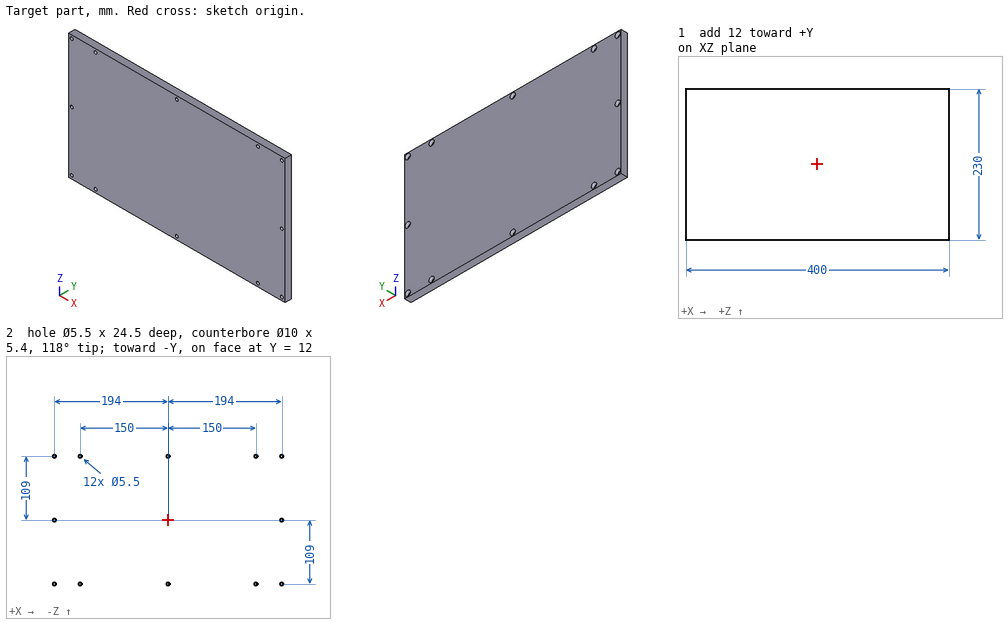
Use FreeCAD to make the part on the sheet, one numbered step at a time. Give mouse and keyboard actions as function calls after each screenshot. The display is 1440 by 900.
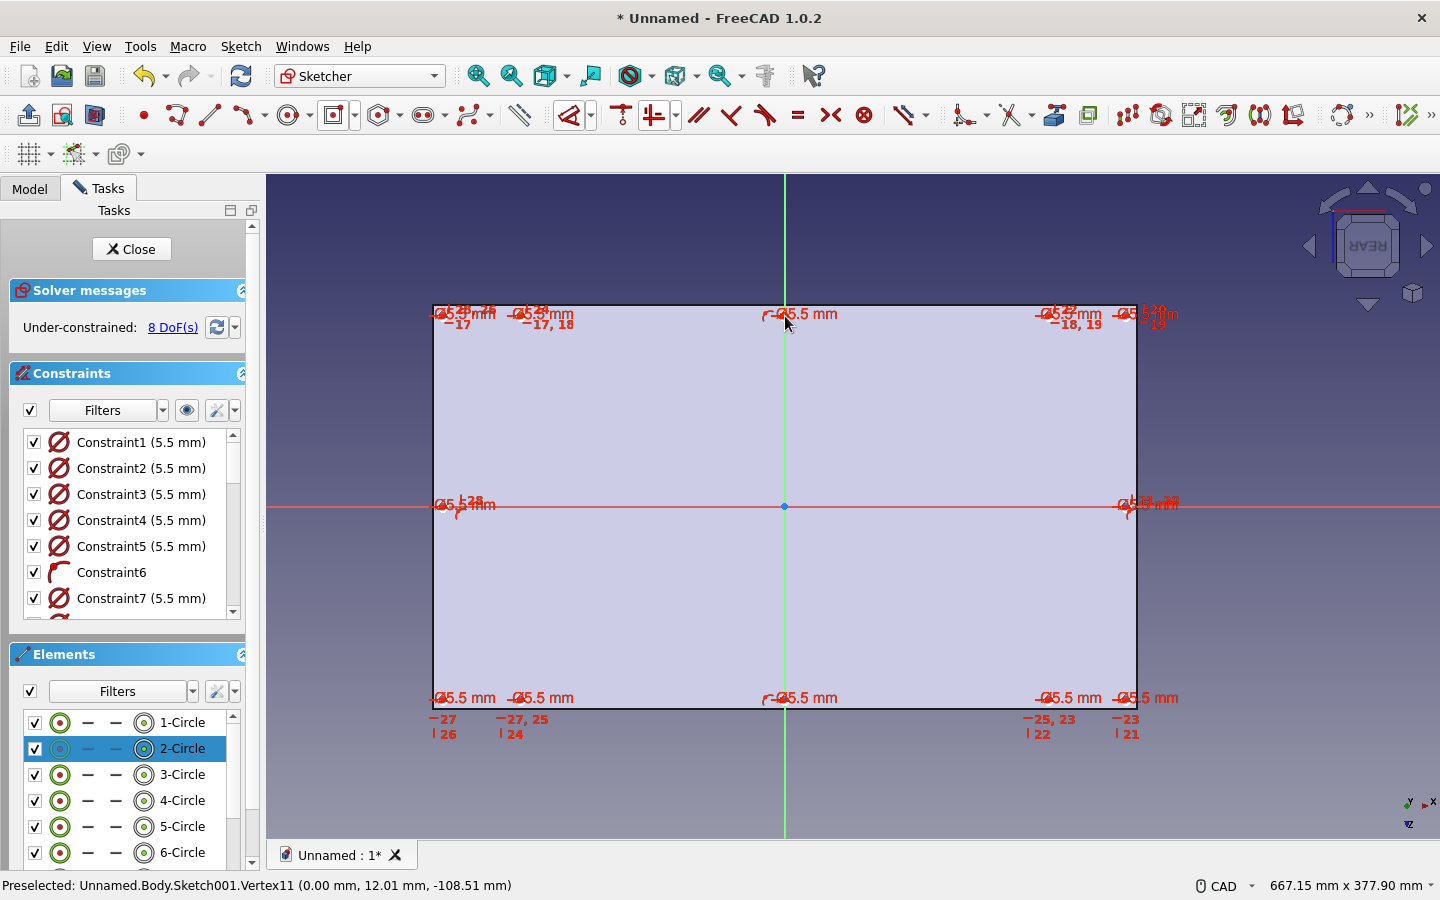
click(676, 116)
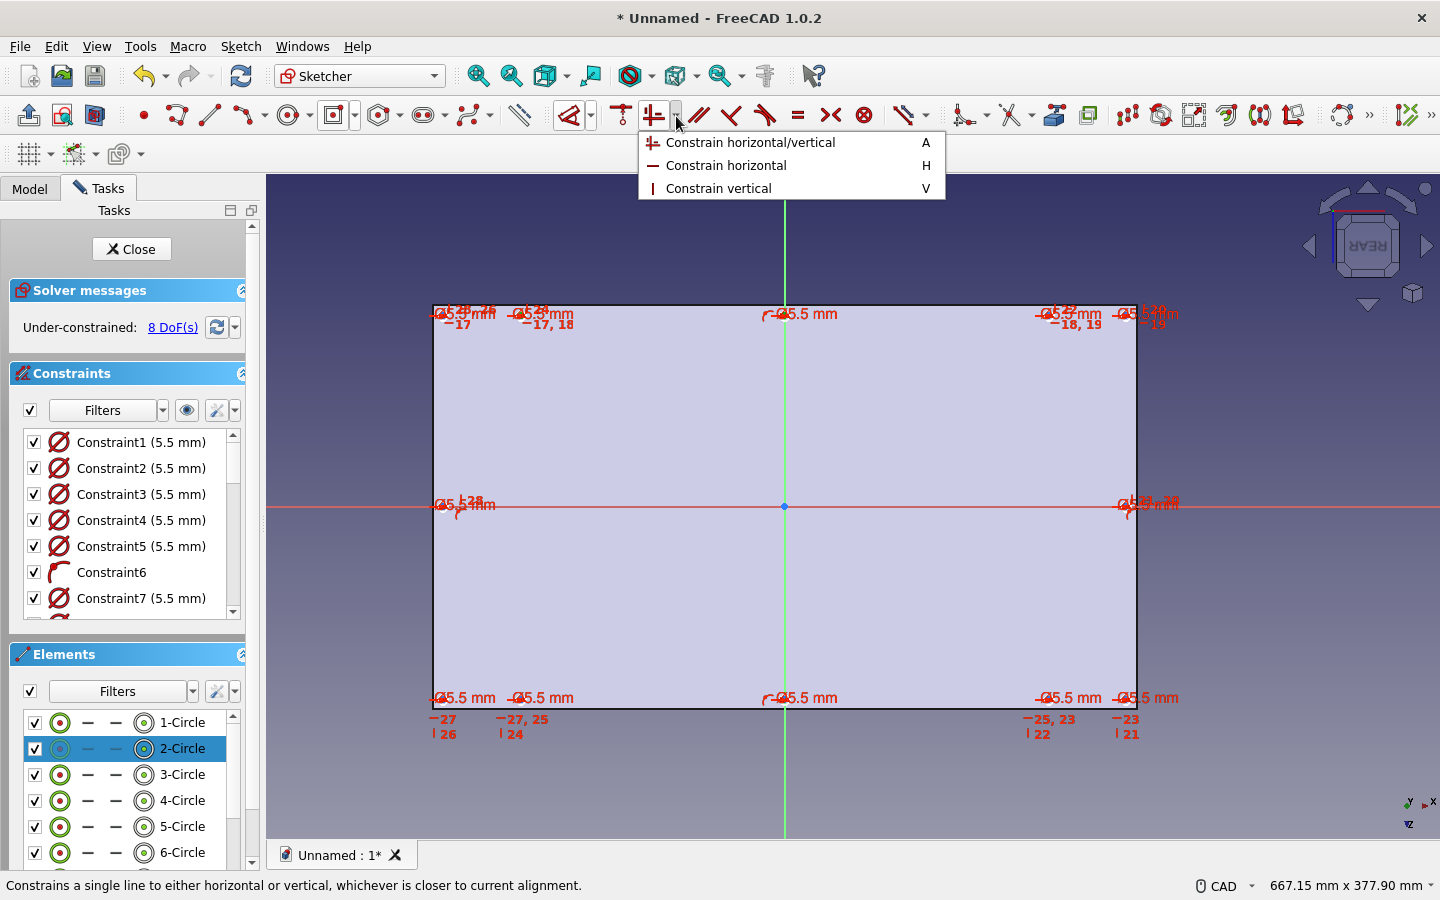
click(792, 166)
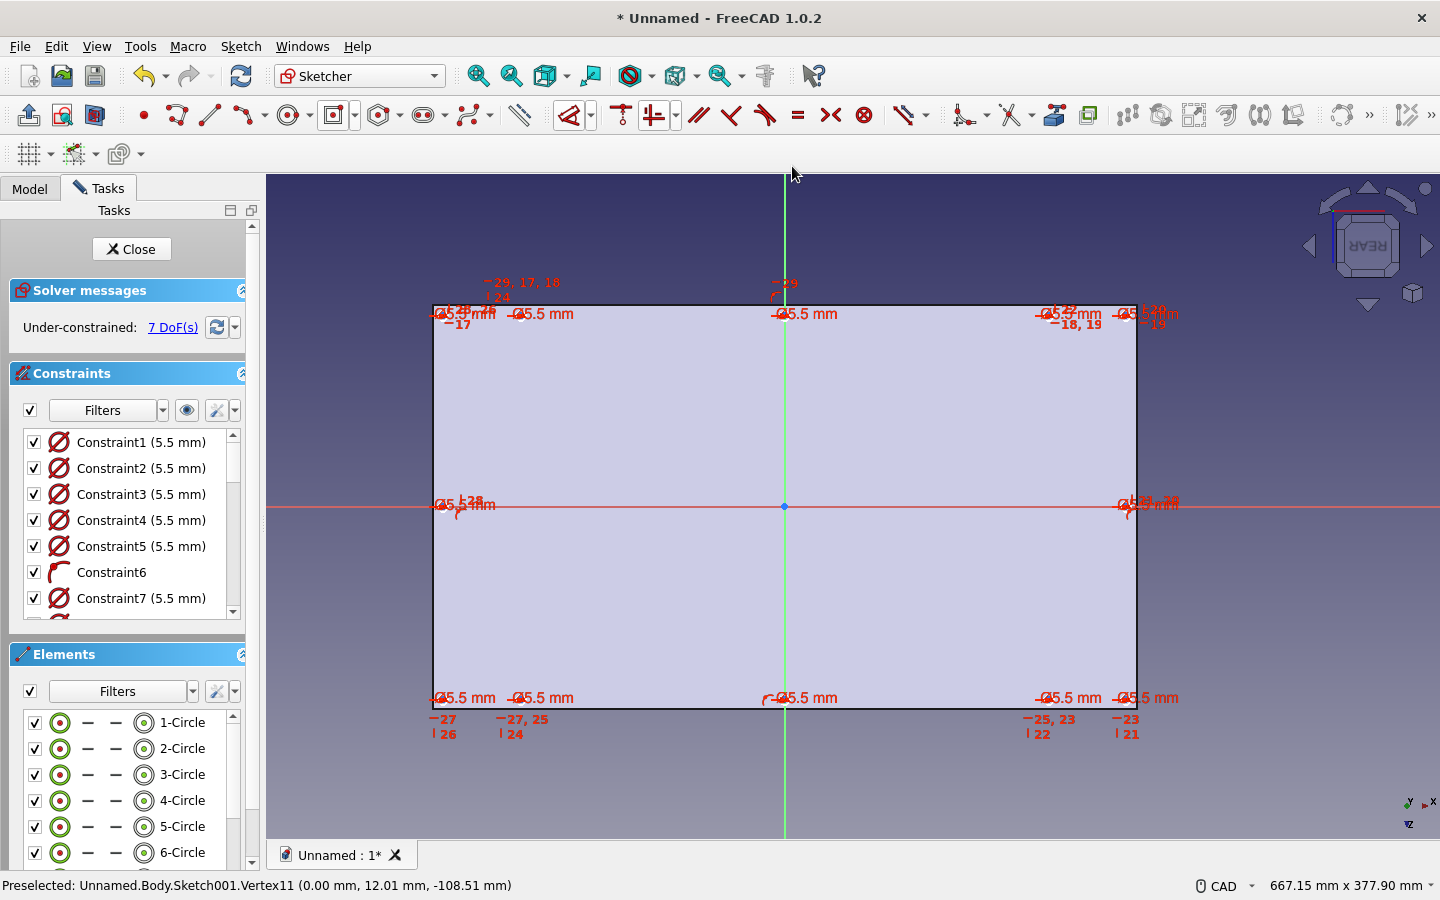
click(1049, 700)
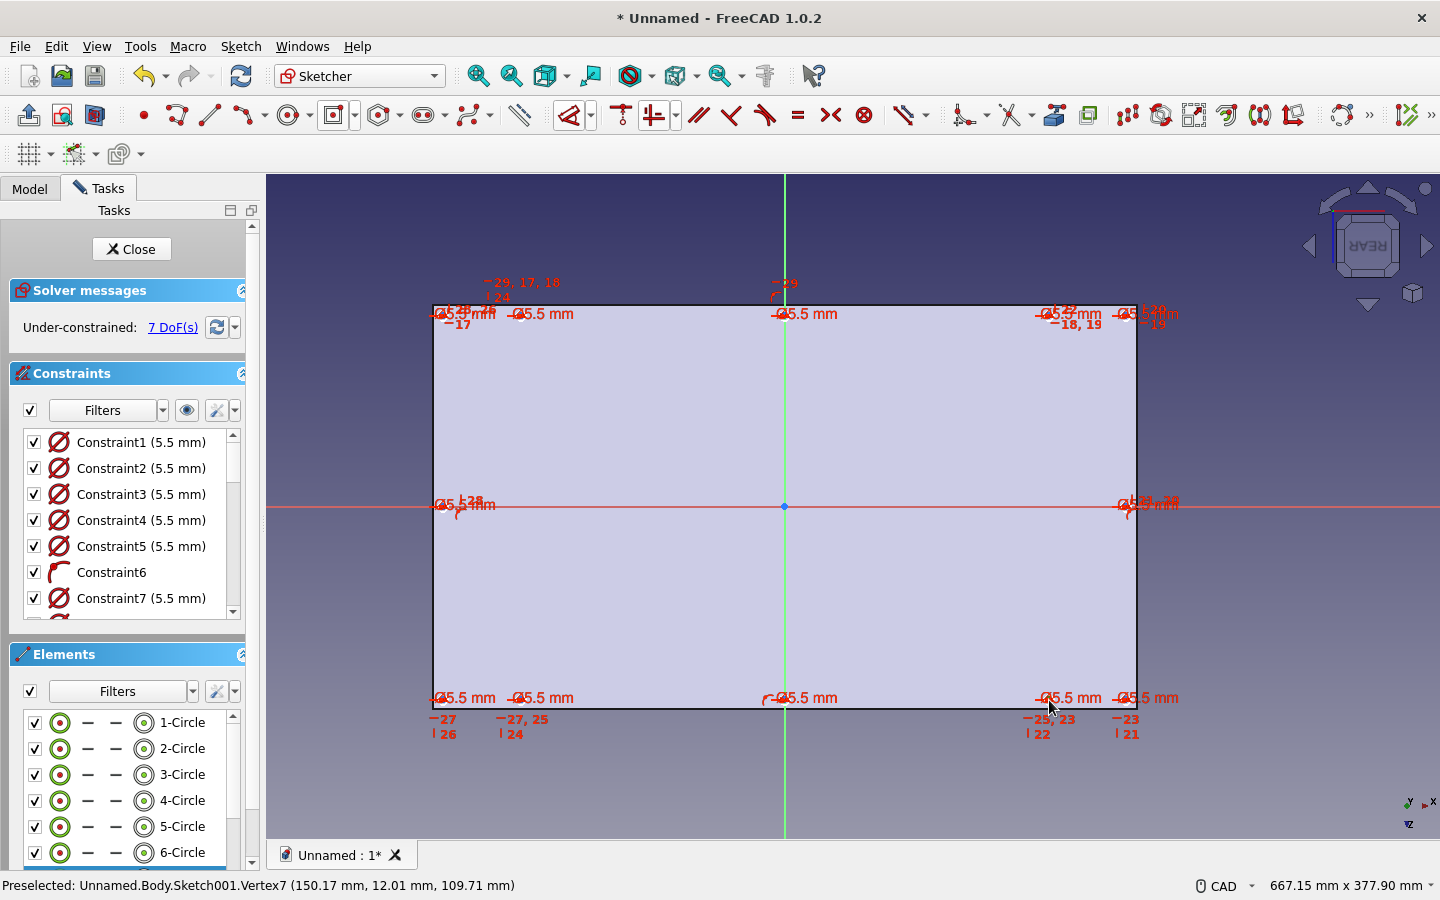
click(785, 700)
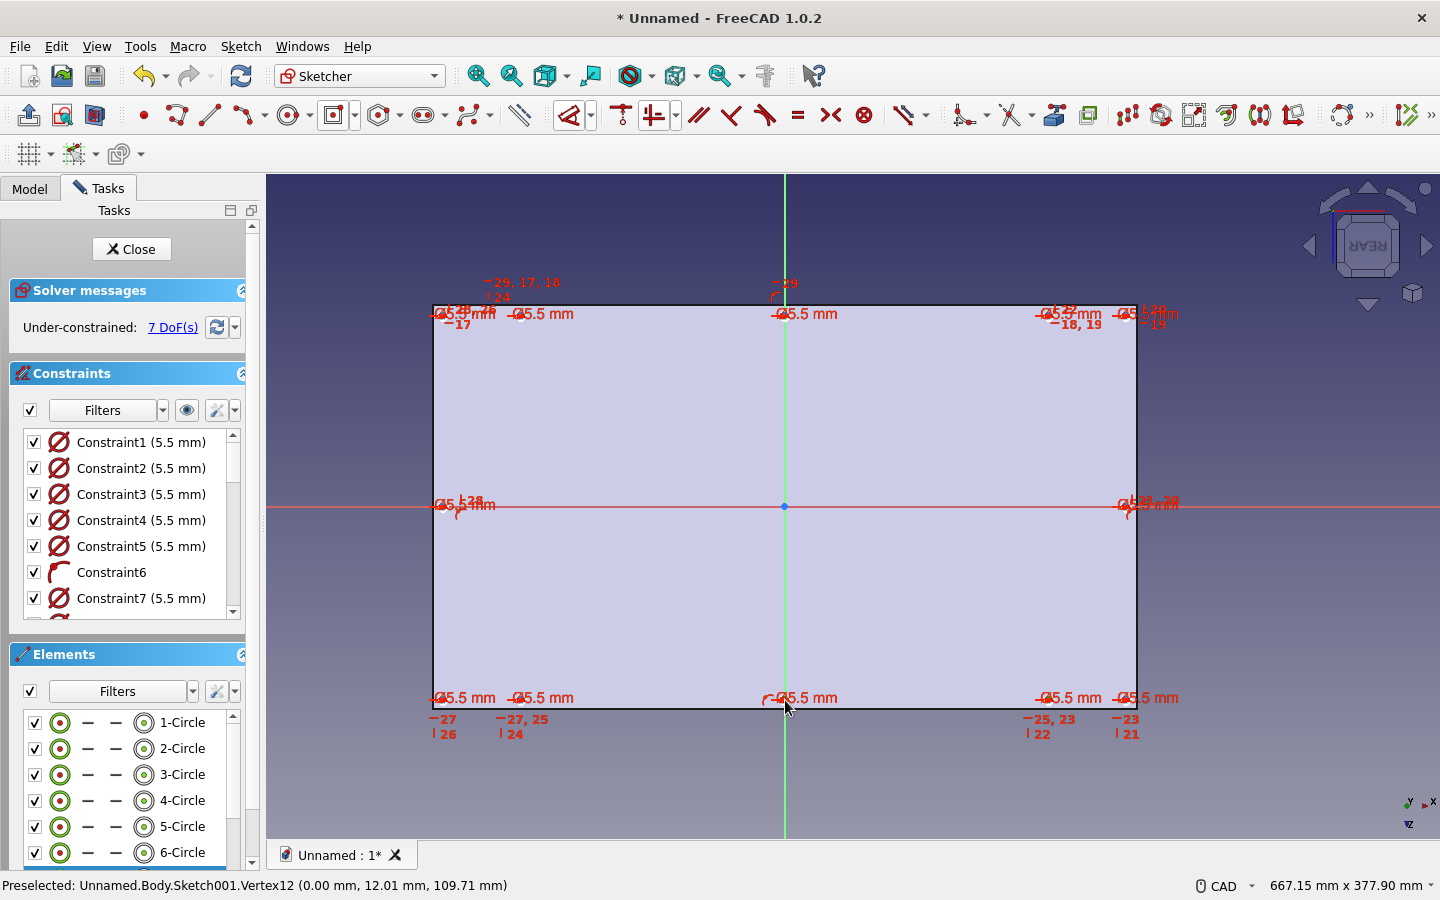
click(676, 116)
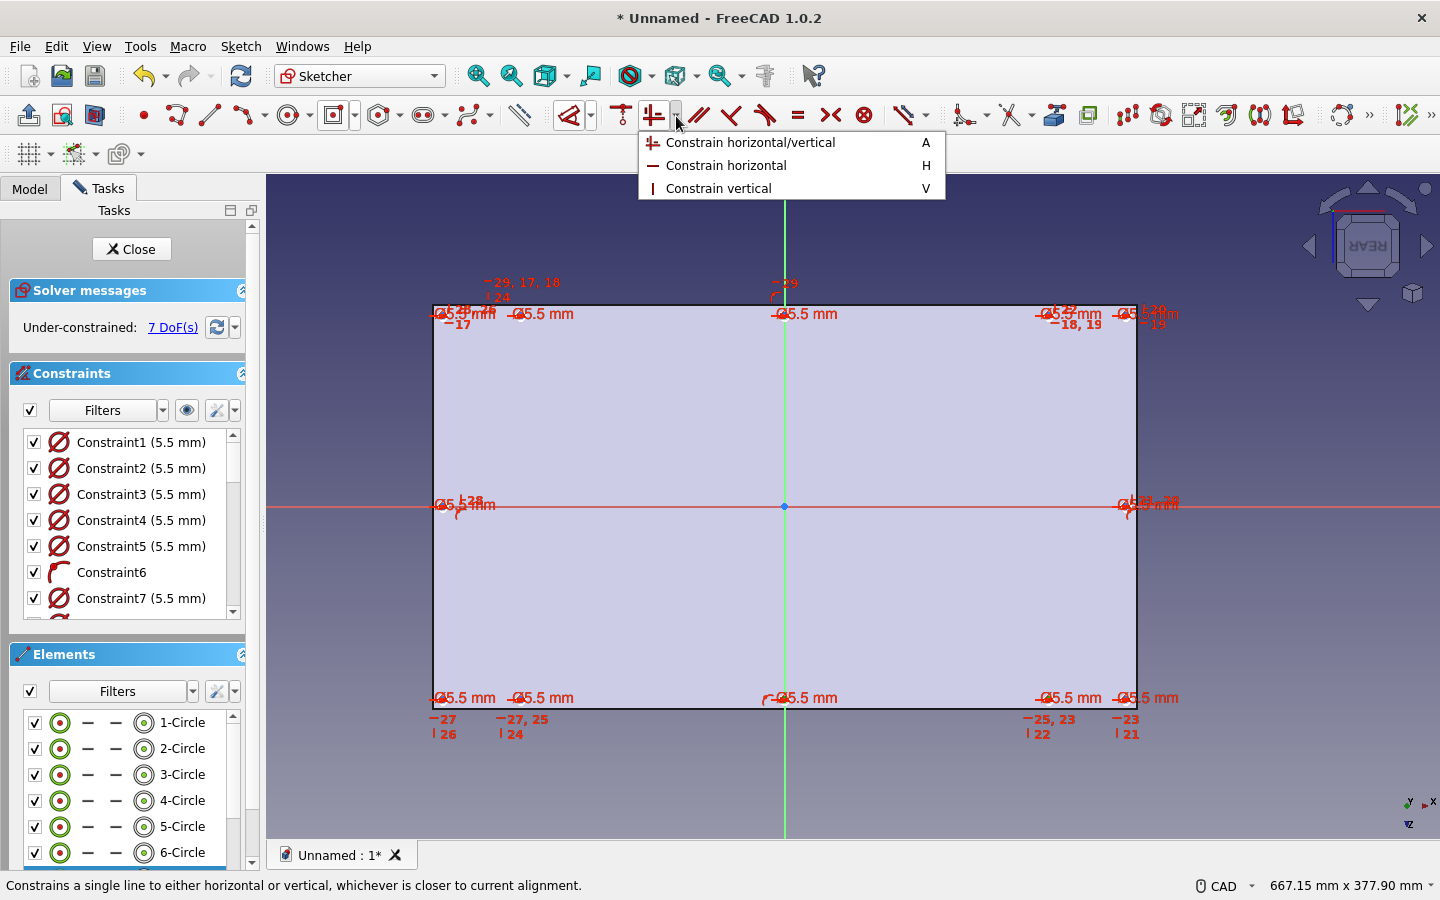
click(792, 166)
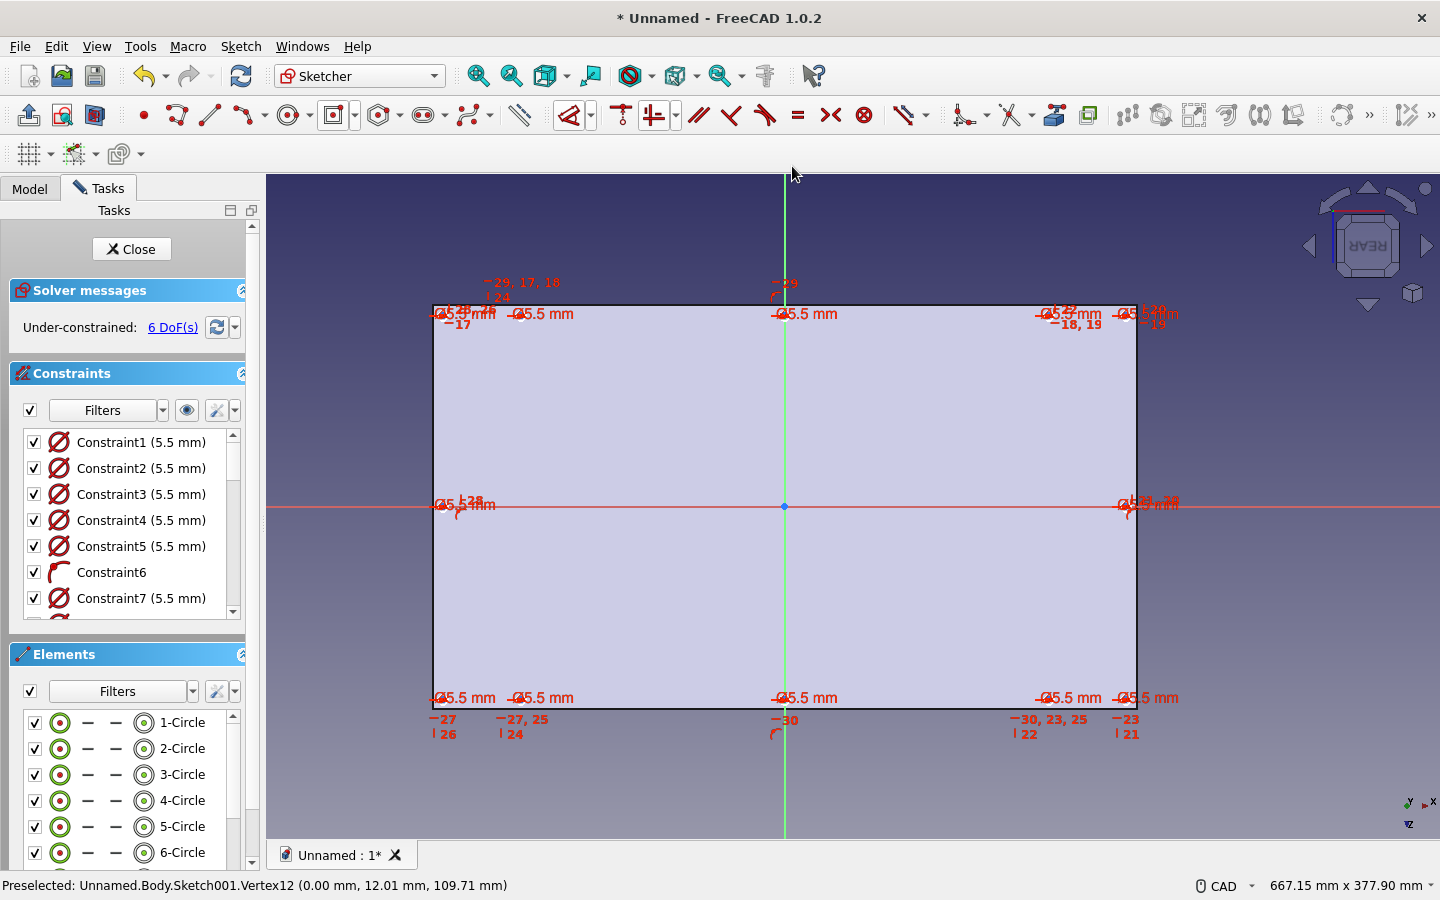
click(443, 316)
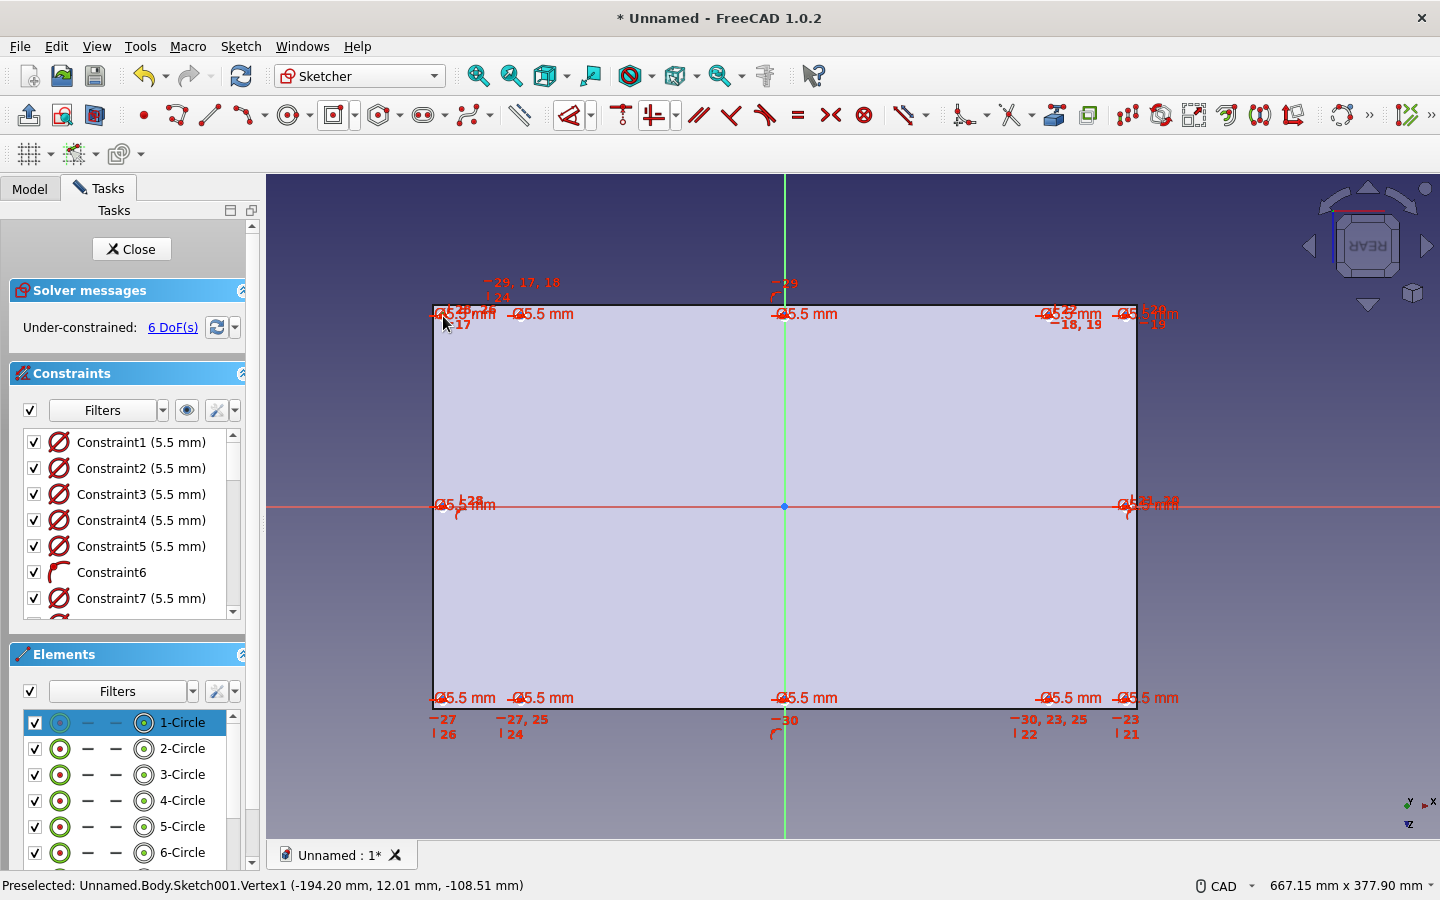
click(590, 116)